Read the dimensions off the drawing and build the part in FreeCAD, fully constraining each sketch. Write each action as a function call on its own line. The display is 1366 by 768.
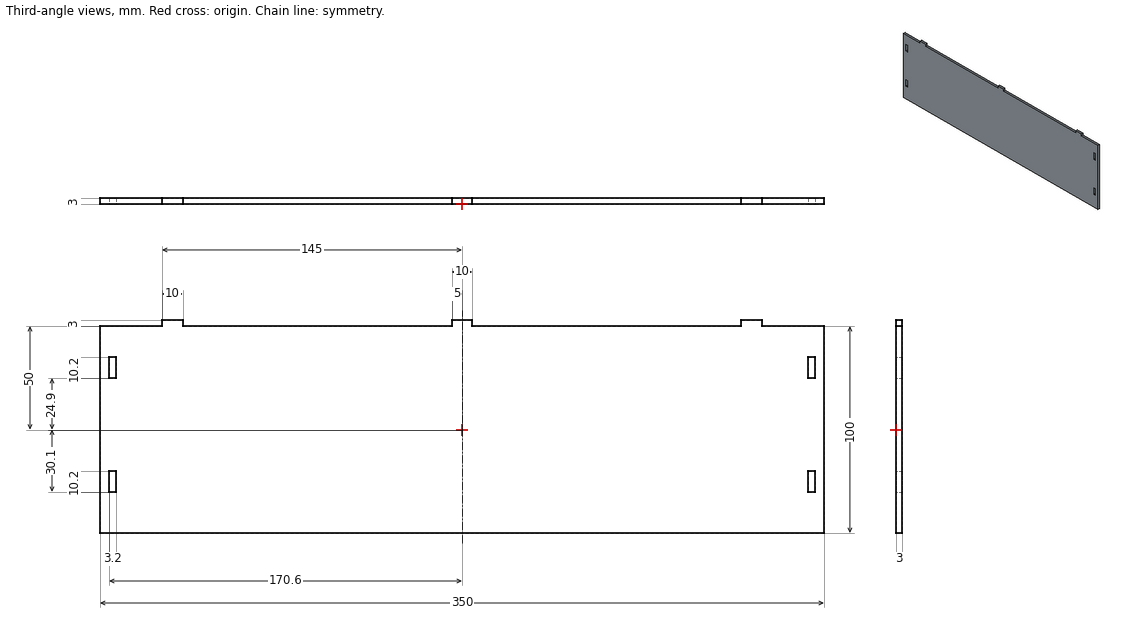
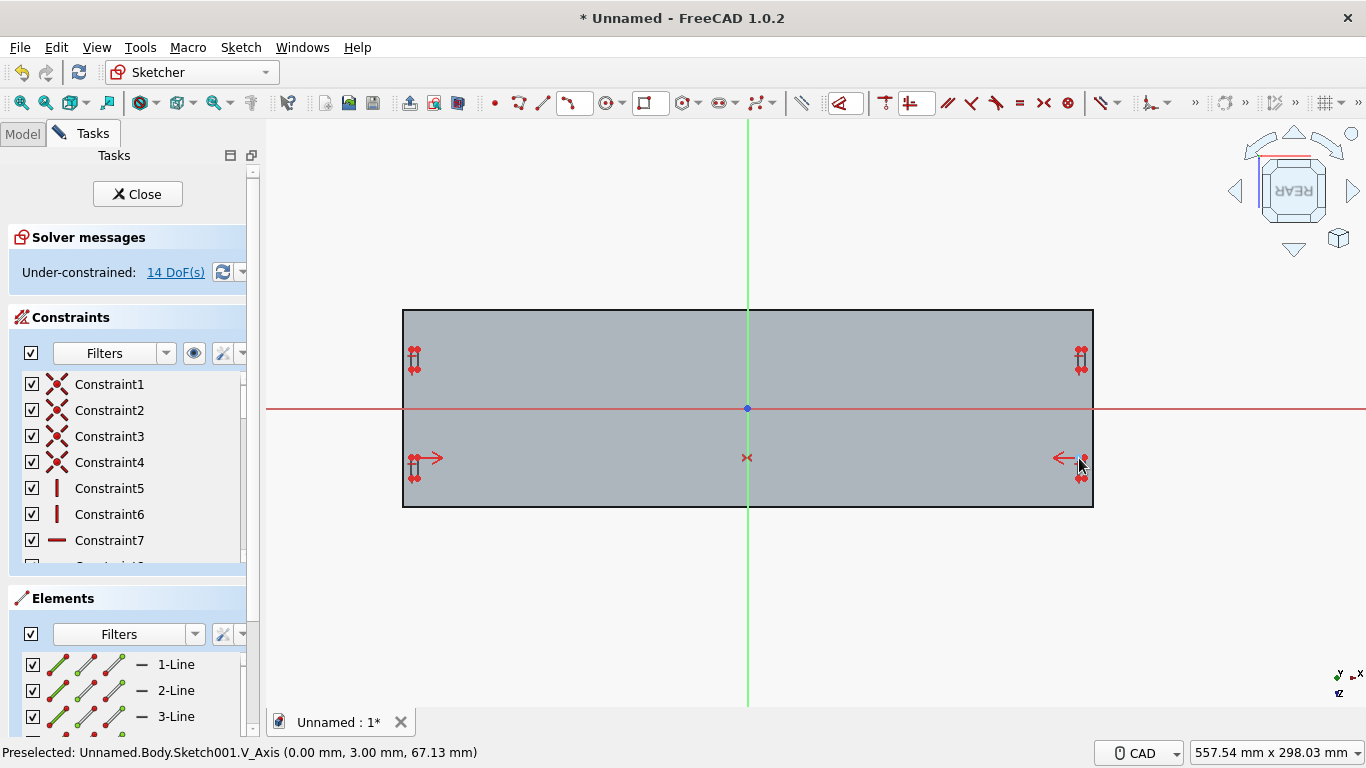
scroll(411, 479, up, 4)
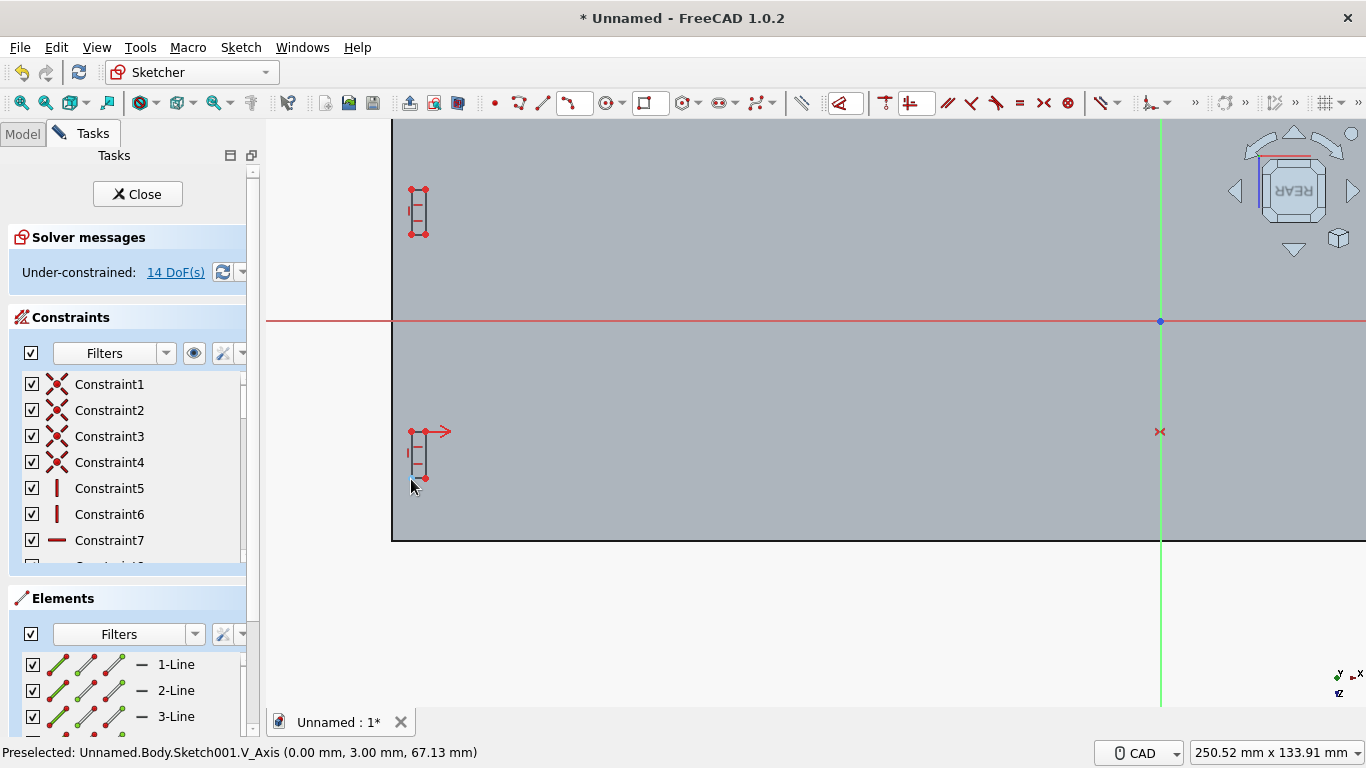
click(412, 478)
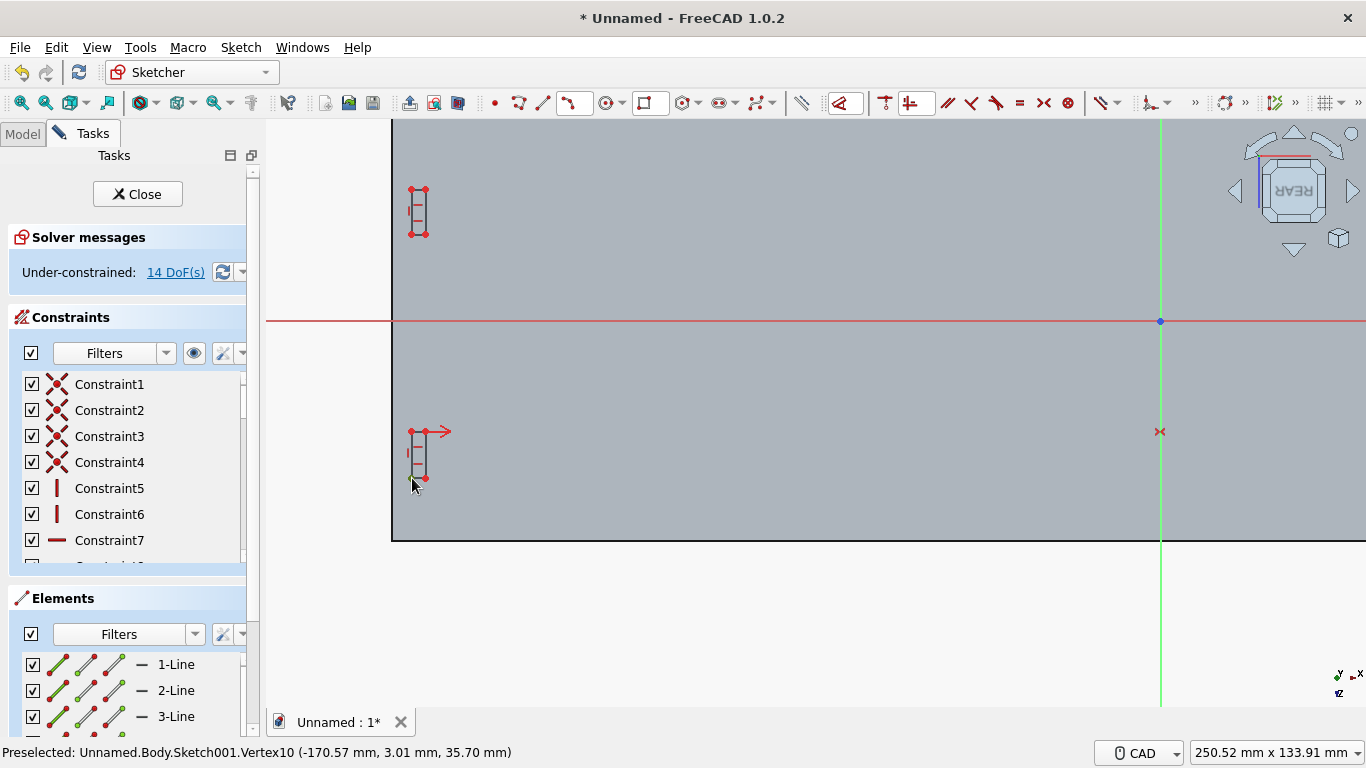
scroll(410, 479, down, 4)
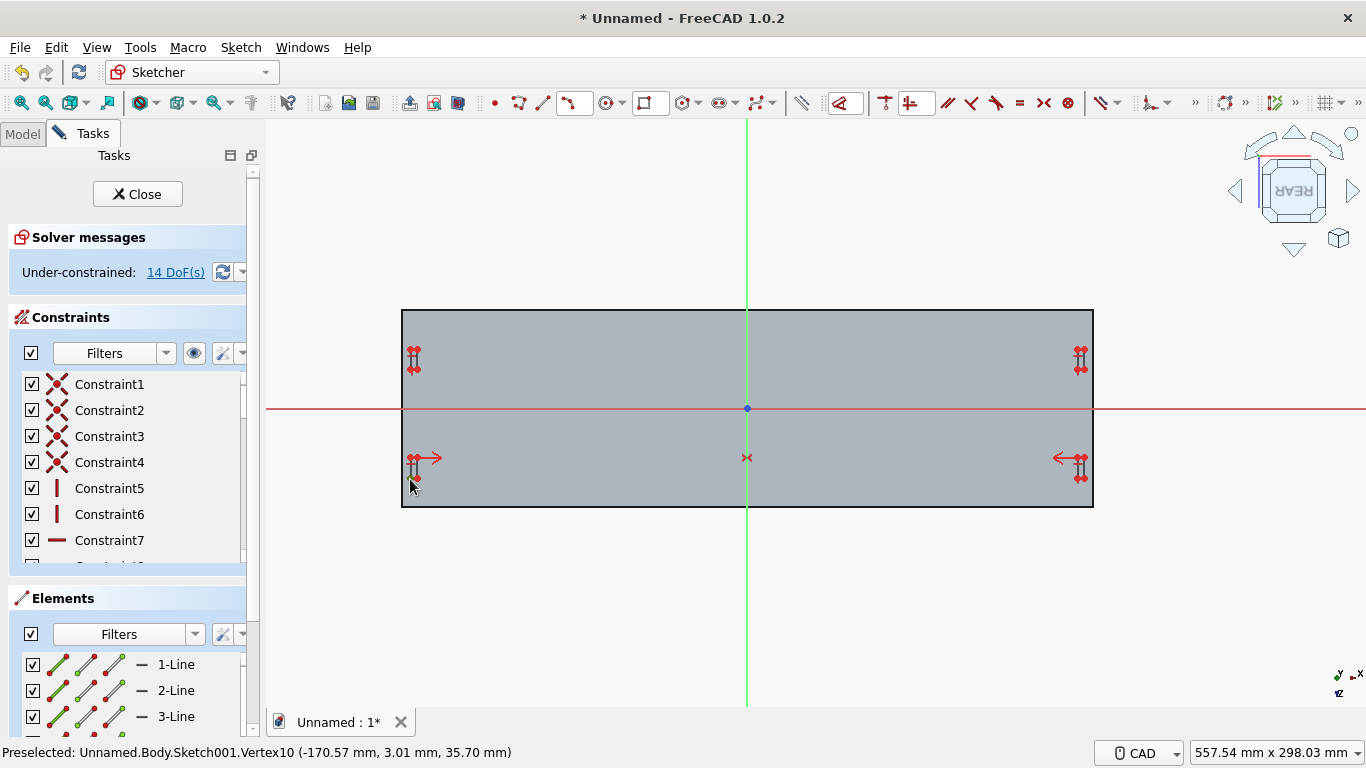
scroll(1084, 478, up, 4)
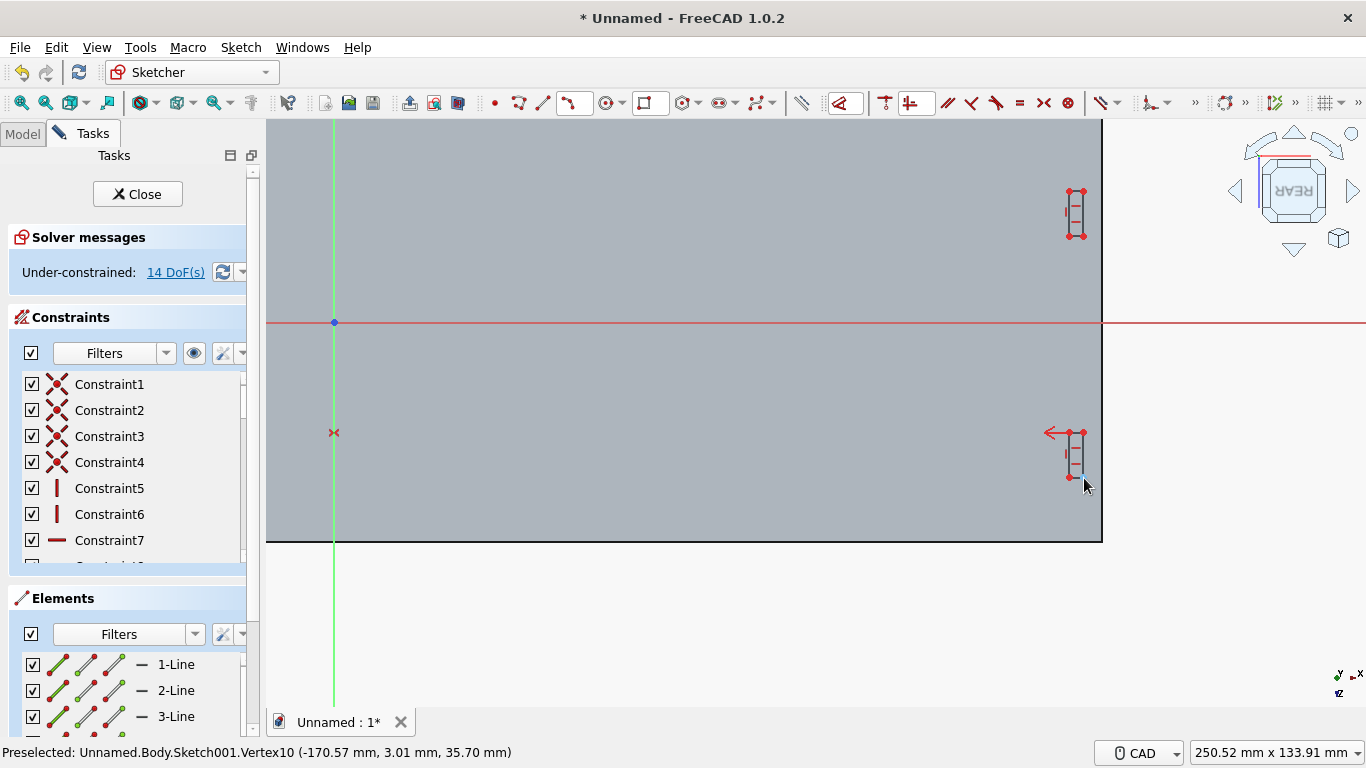
click(1083, 478)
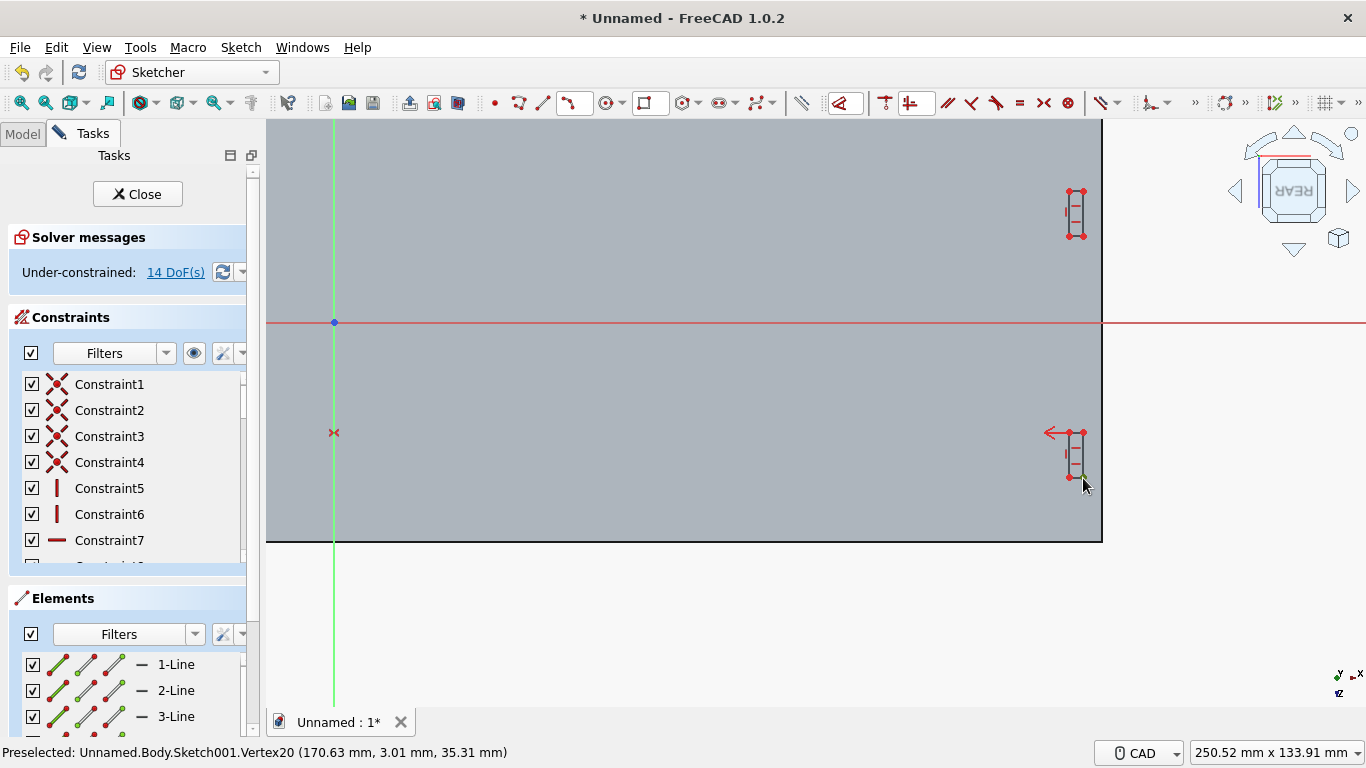
click(334, 641)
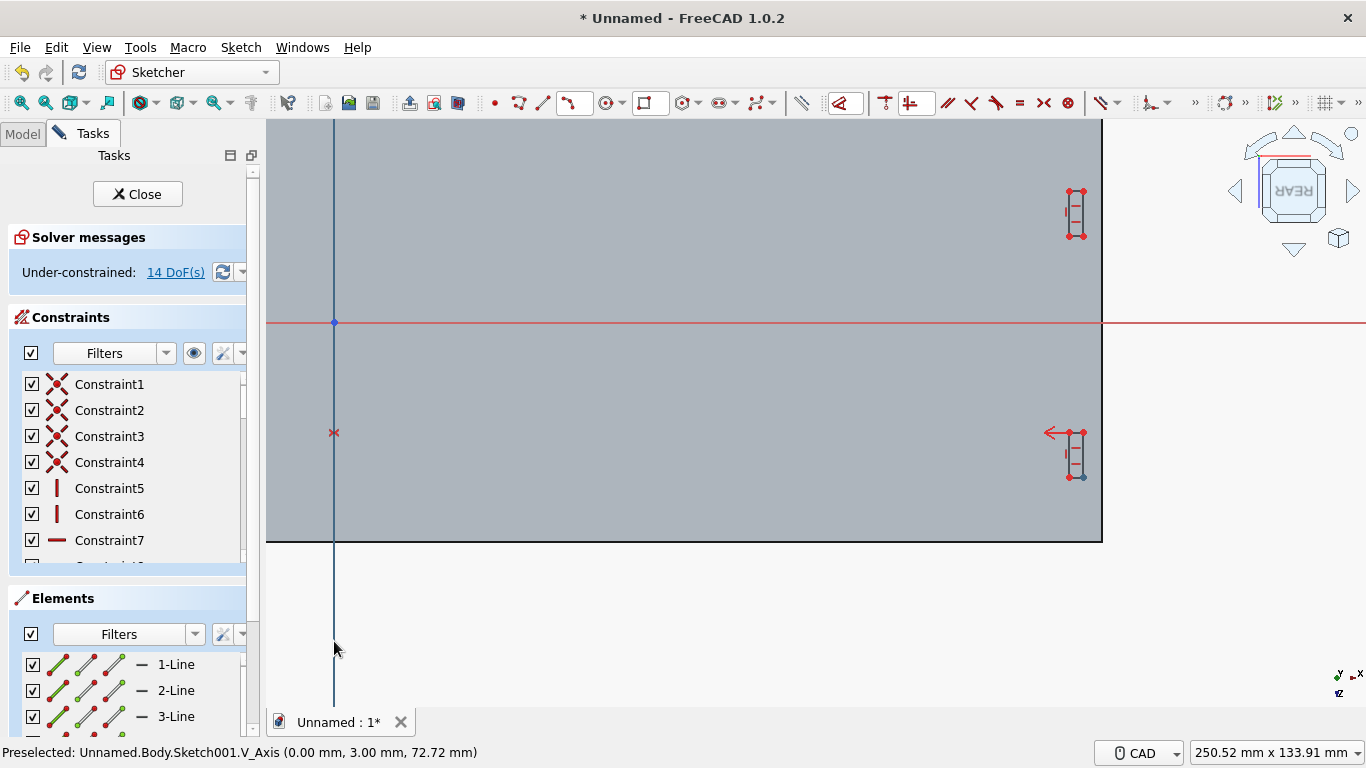
click(1044, 104)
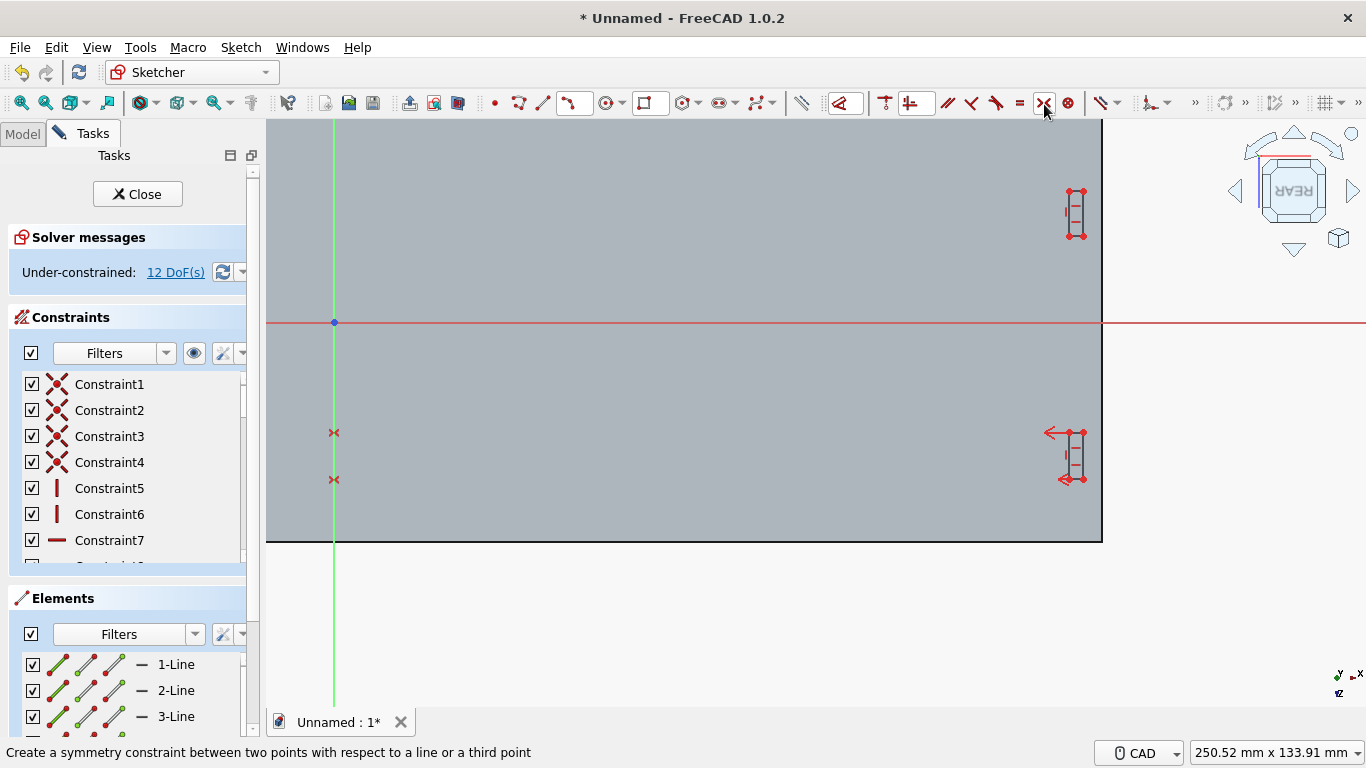
scroll(1085, 478, down, 4)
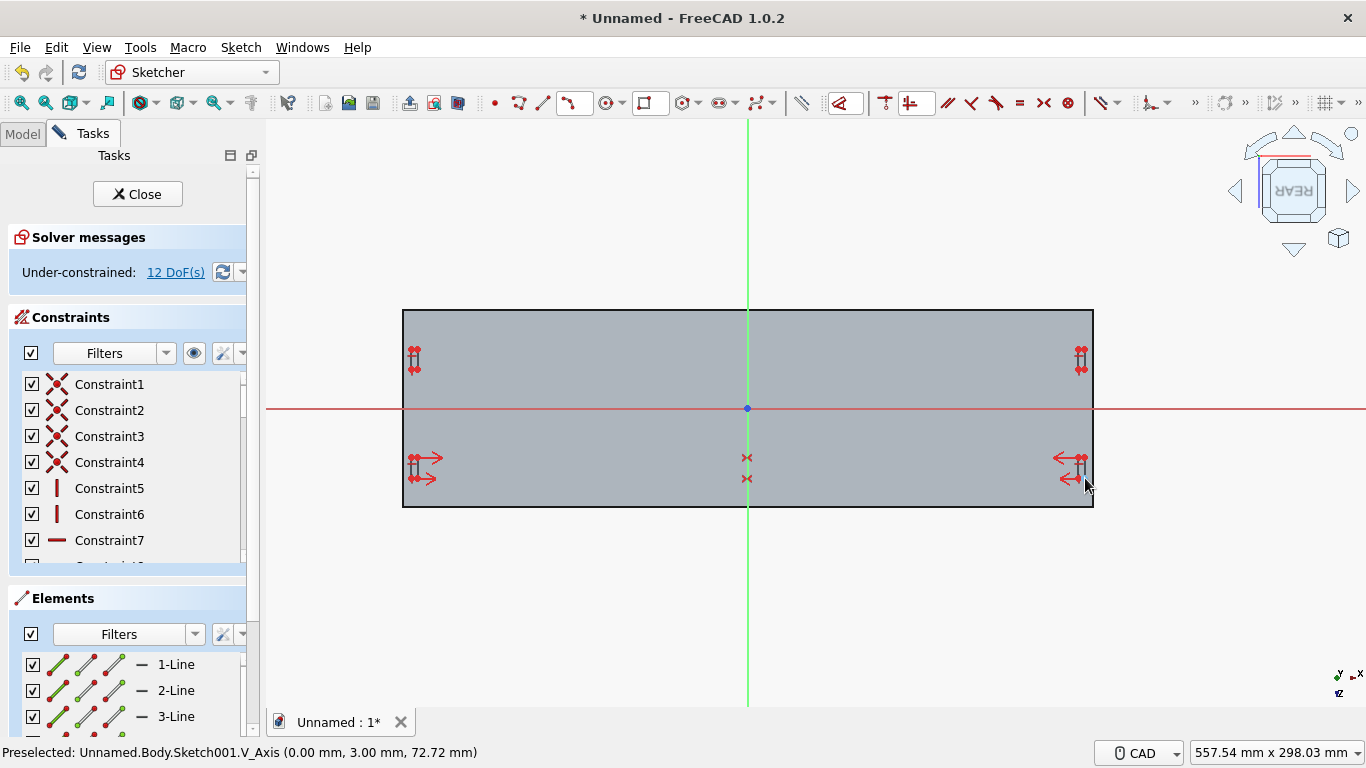
scroll(418, 349, up, 4)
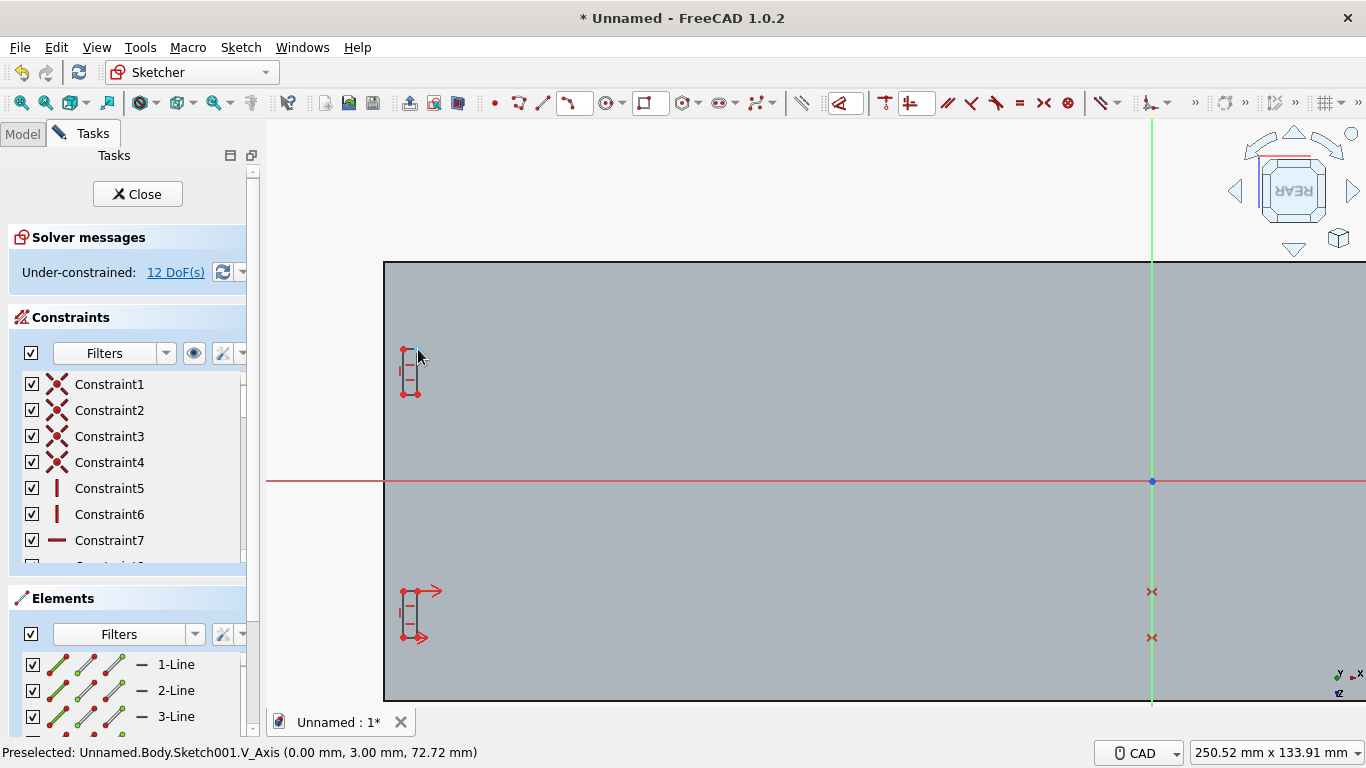
click(417, 349)